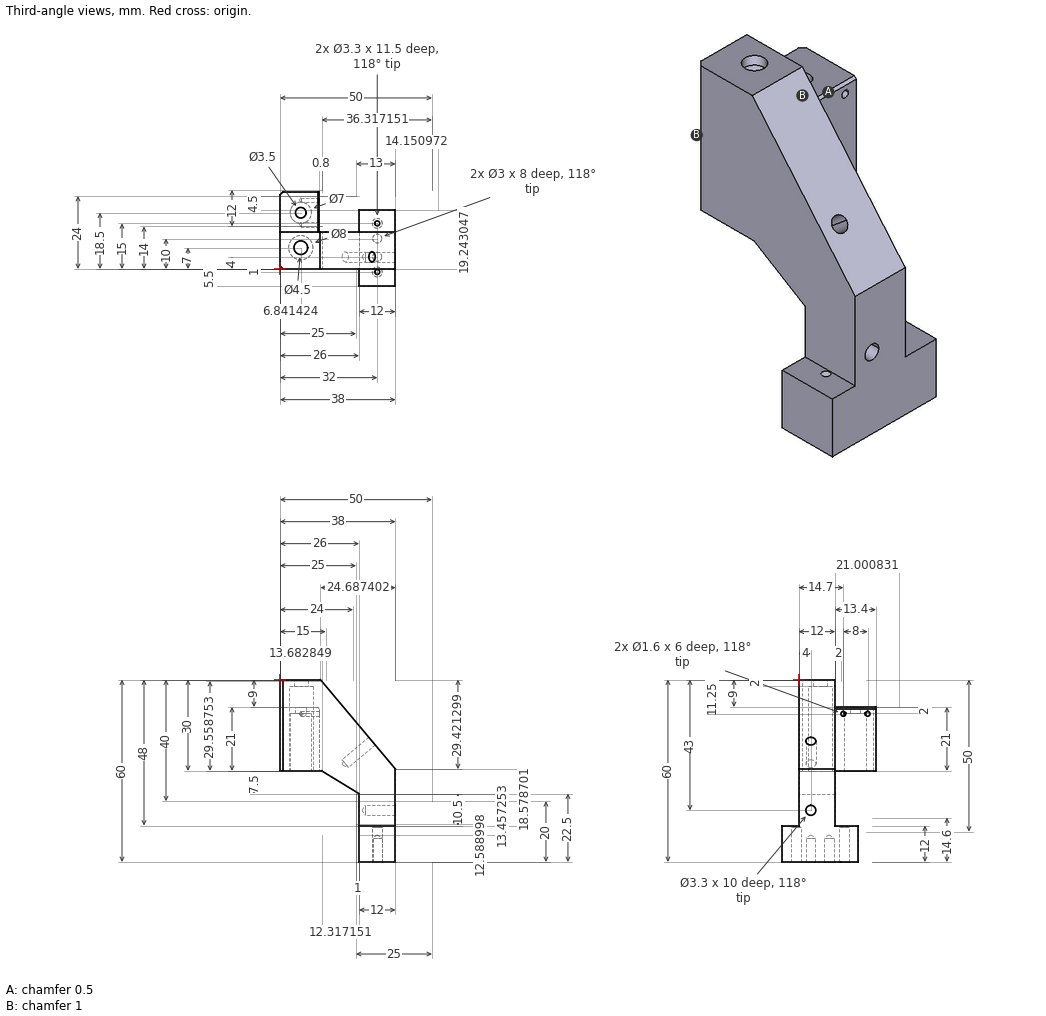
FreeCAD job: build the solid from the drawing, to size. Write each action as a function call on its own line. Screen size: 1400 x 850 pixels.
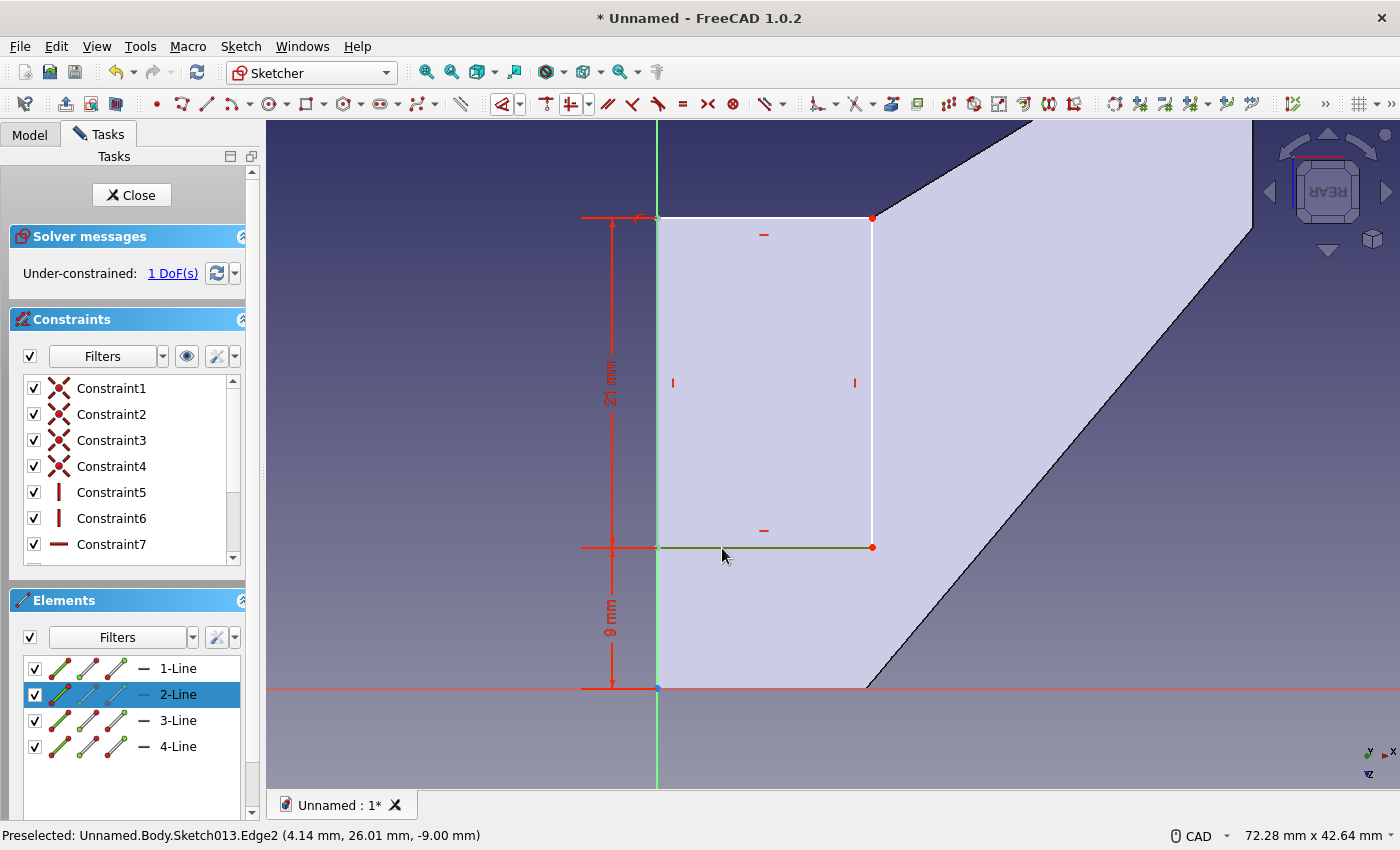
click(520, 104)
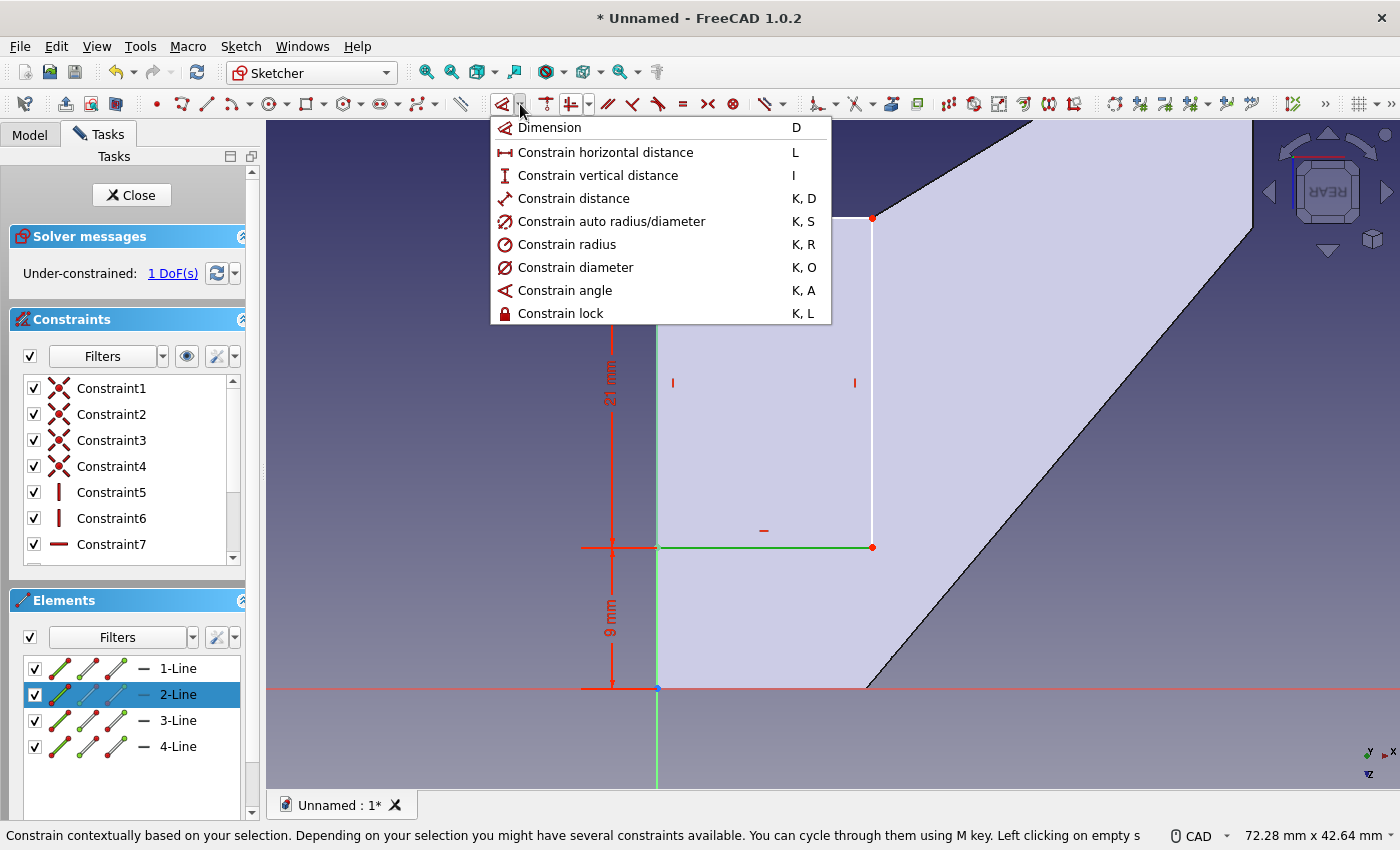
click(661, 152)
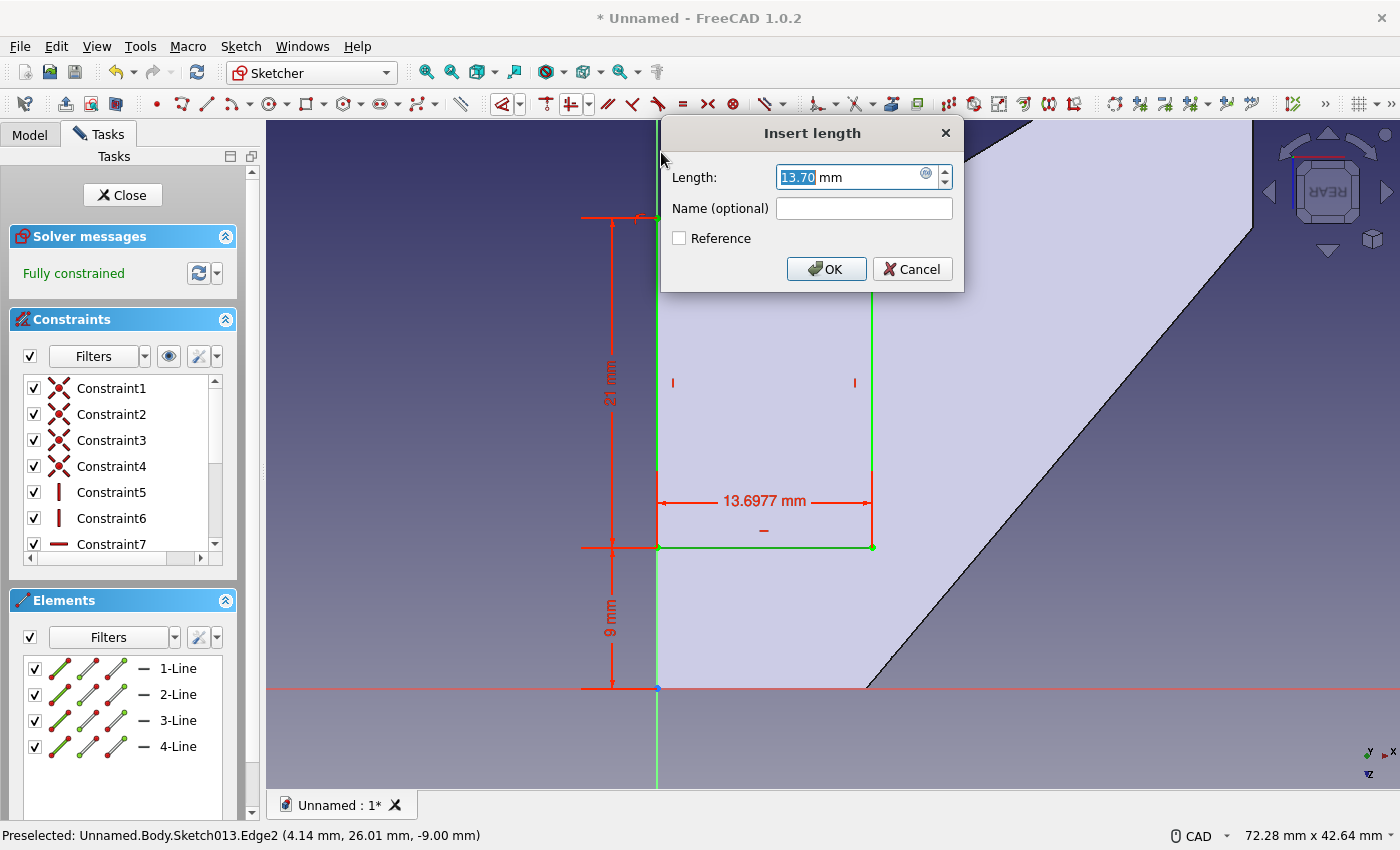
text(13.682849)
key(Return)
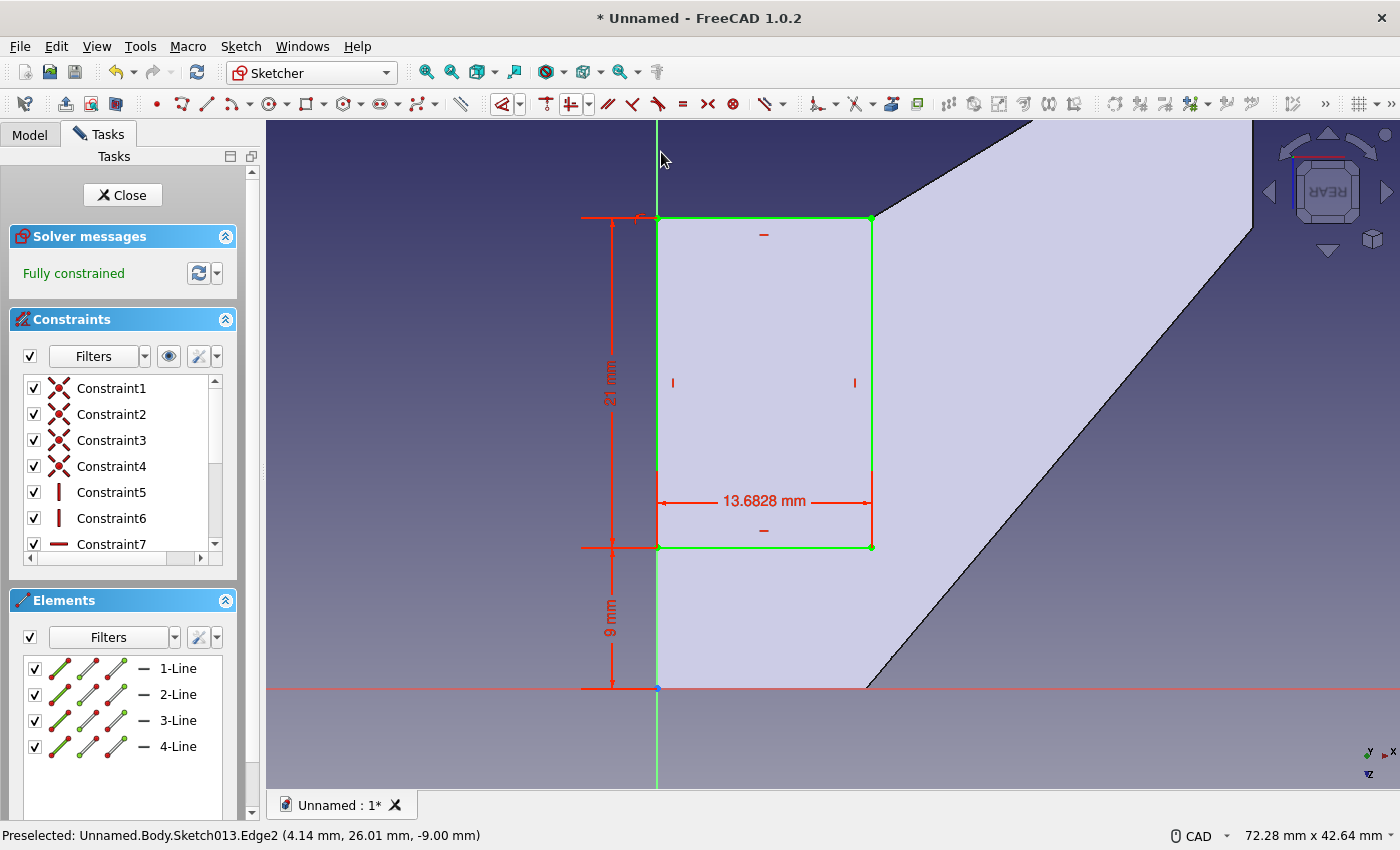
click(123, 195)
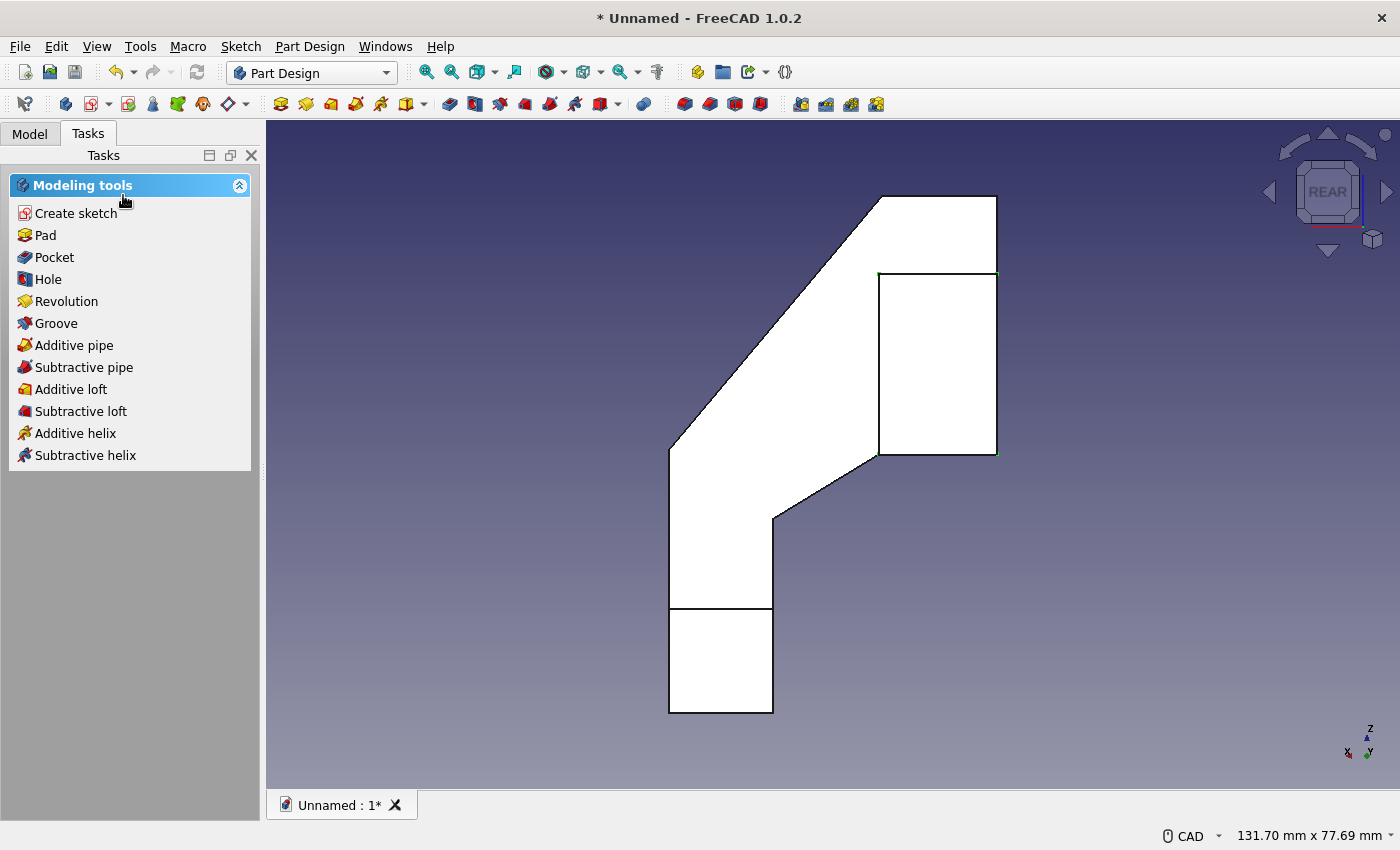
click(450, 104)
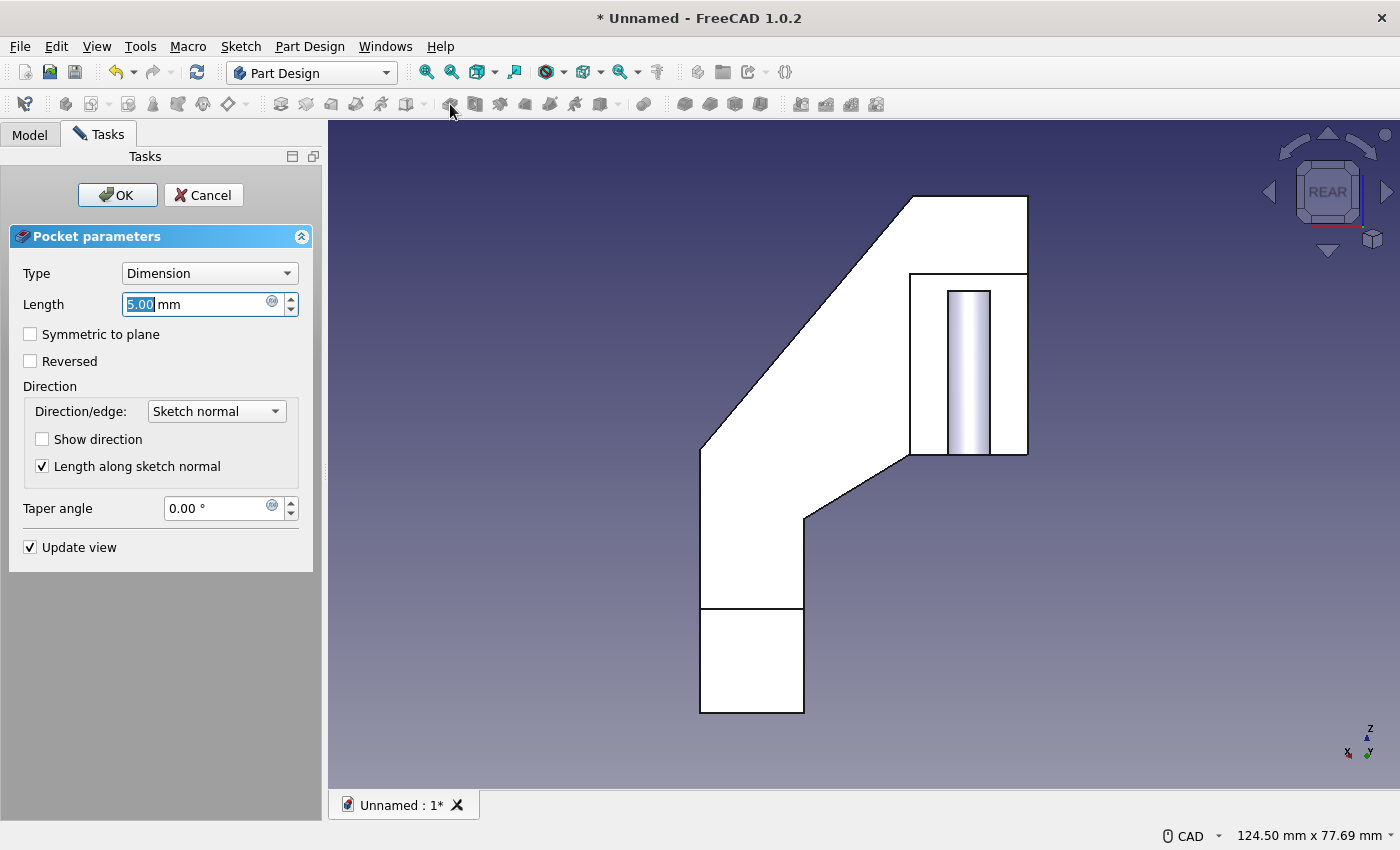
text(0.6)
key(Tab)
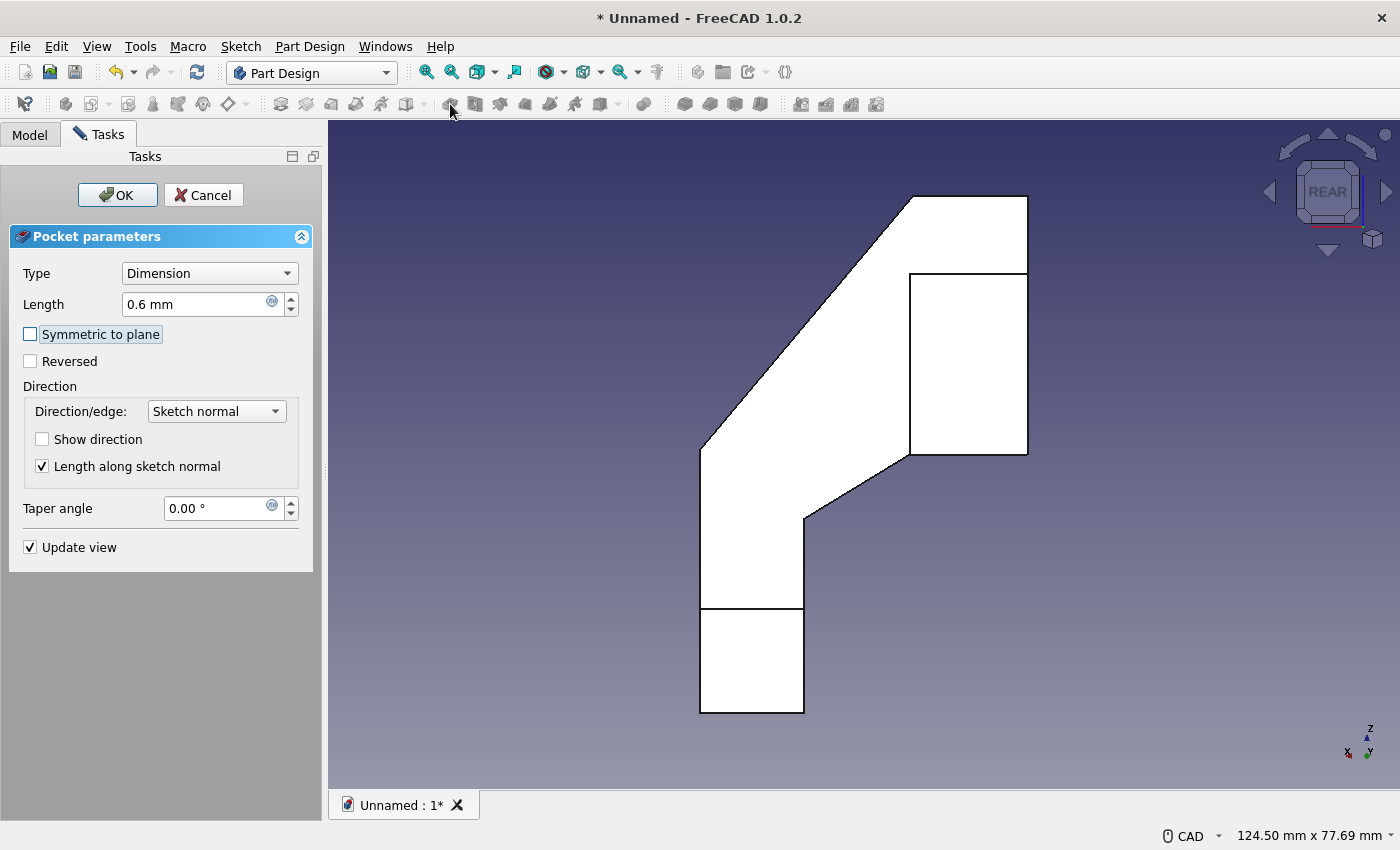
click(118, 195)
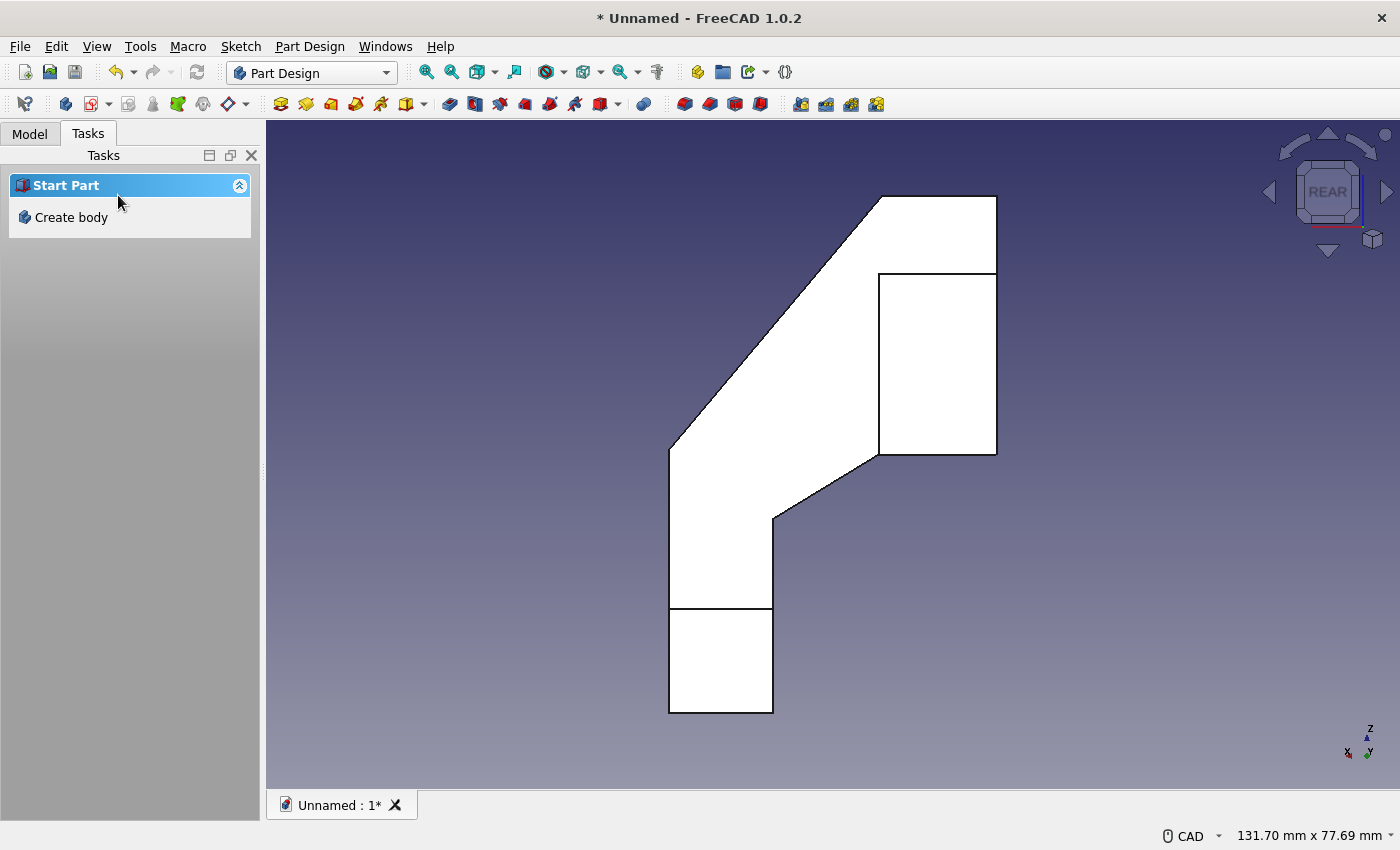
key(0)